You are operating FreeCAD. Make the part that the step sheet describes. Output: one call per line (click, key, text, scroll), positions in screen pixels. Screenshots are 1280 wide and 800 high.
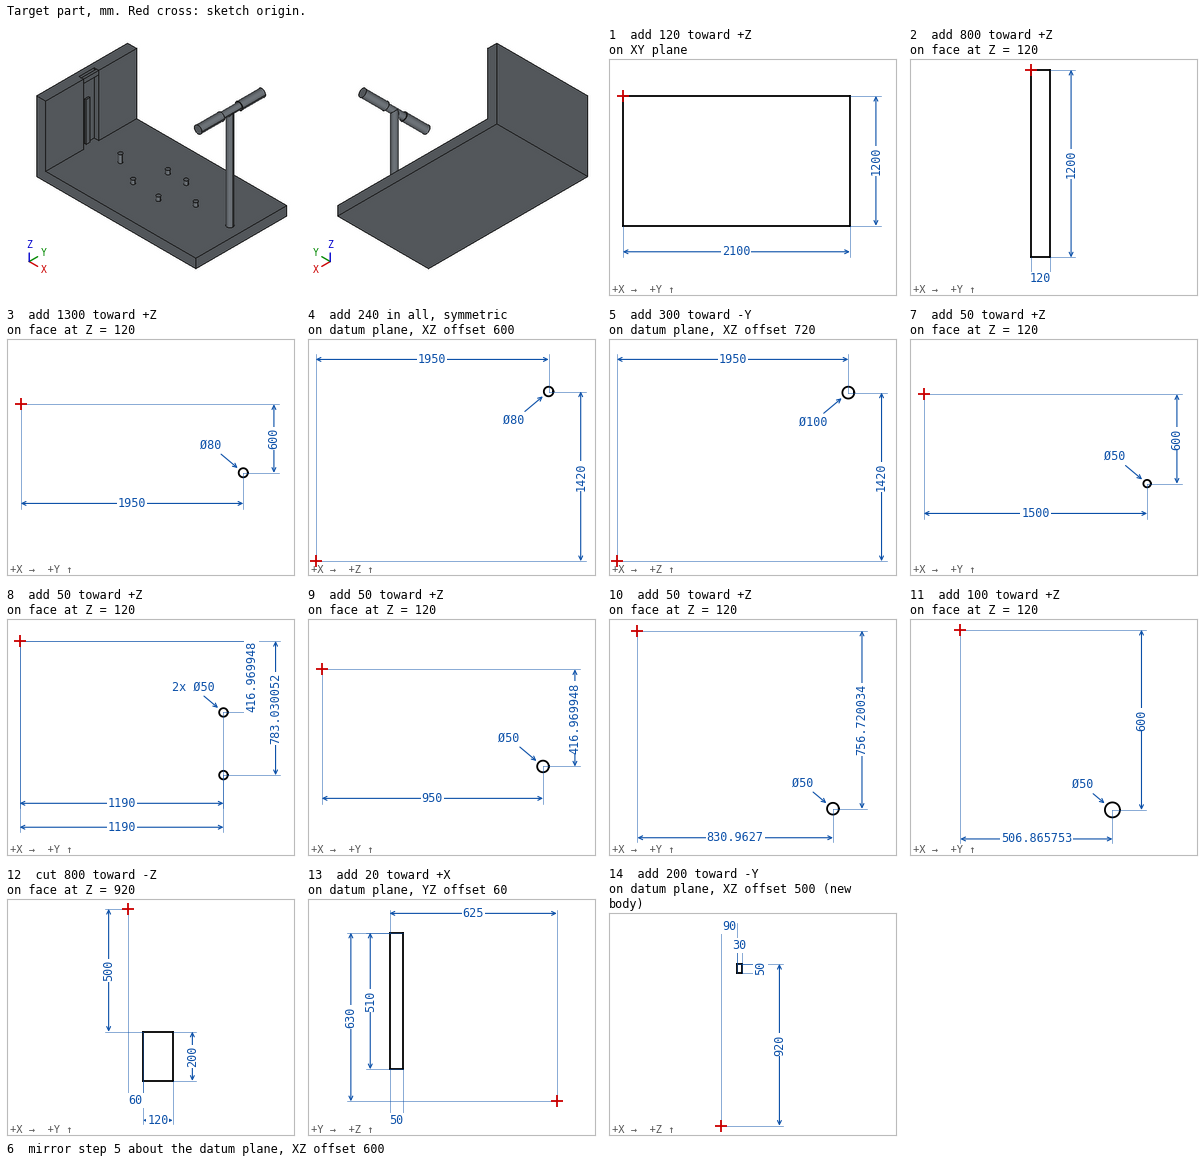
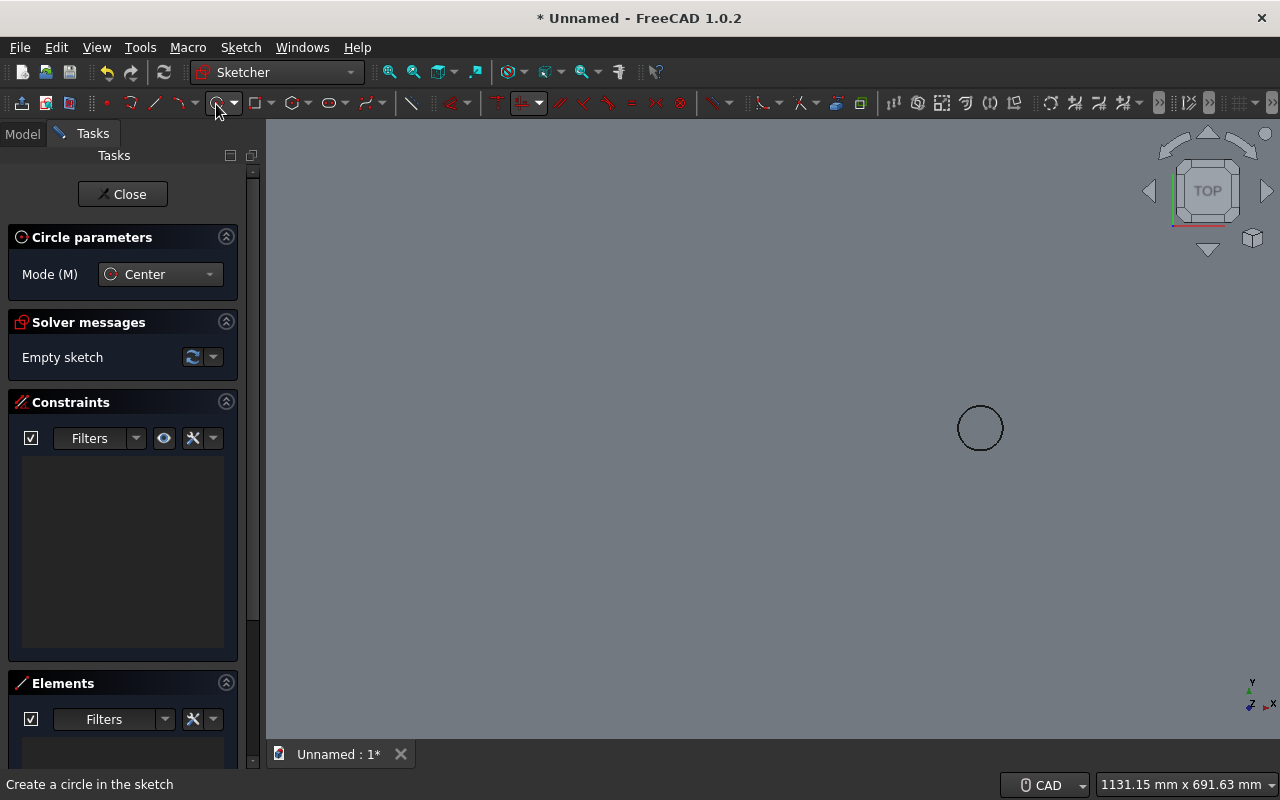
click(703, 264)
move(718, 248)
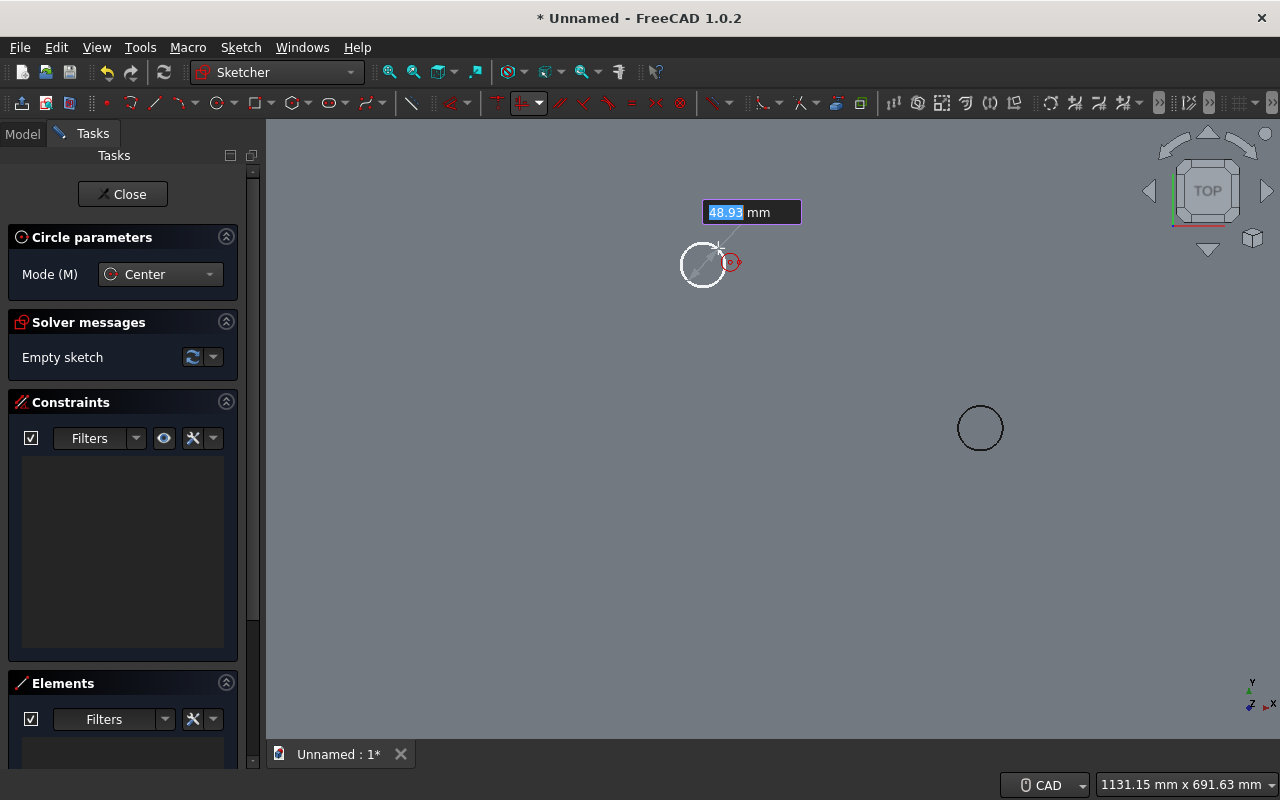
text(50)
key(Return)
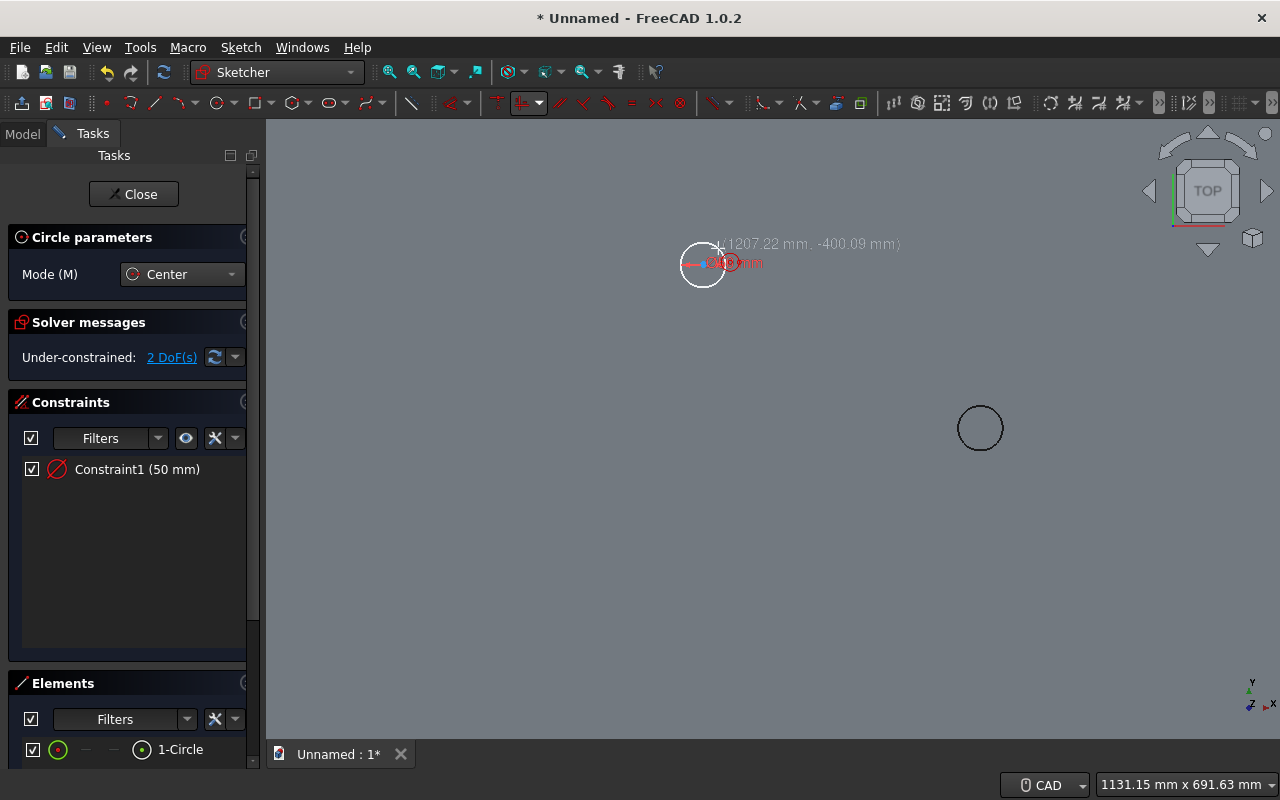
click(703, 592)
move(718, 576)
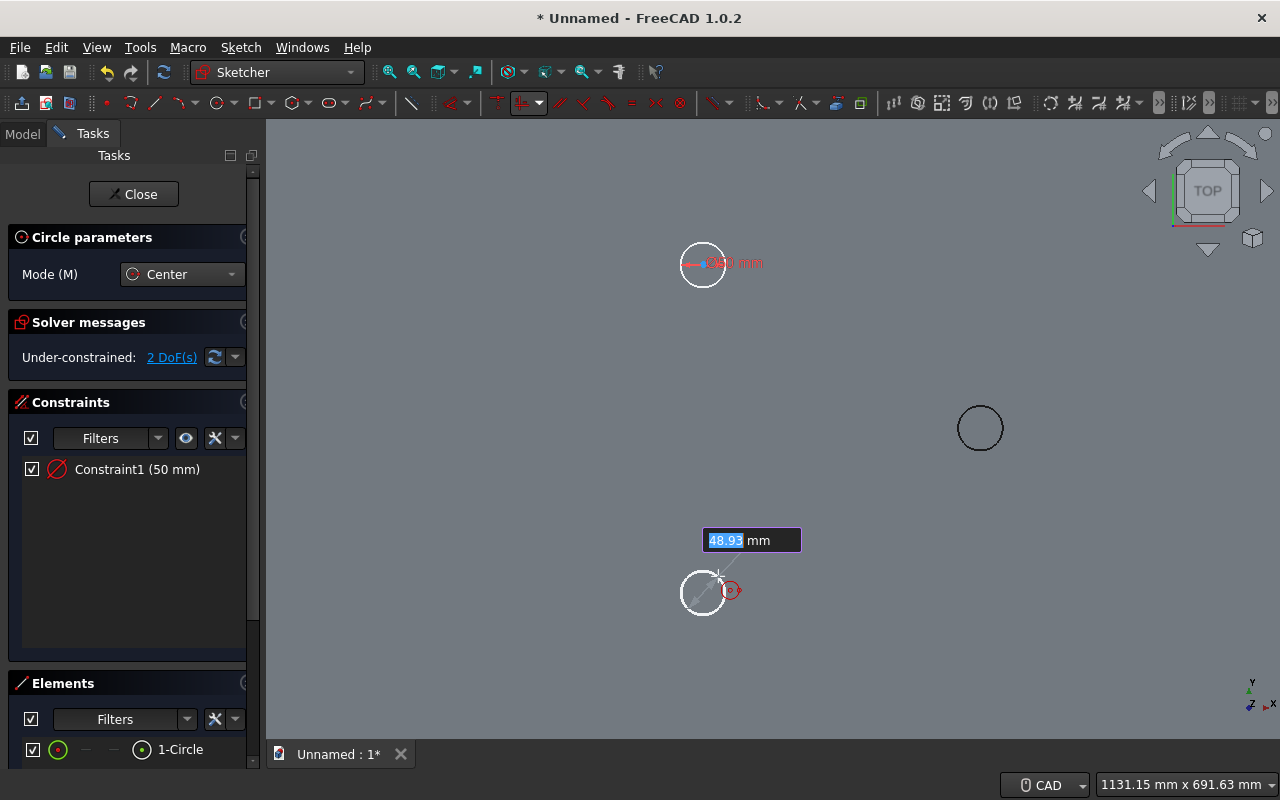
text(50)
key(Return)
key(Escape)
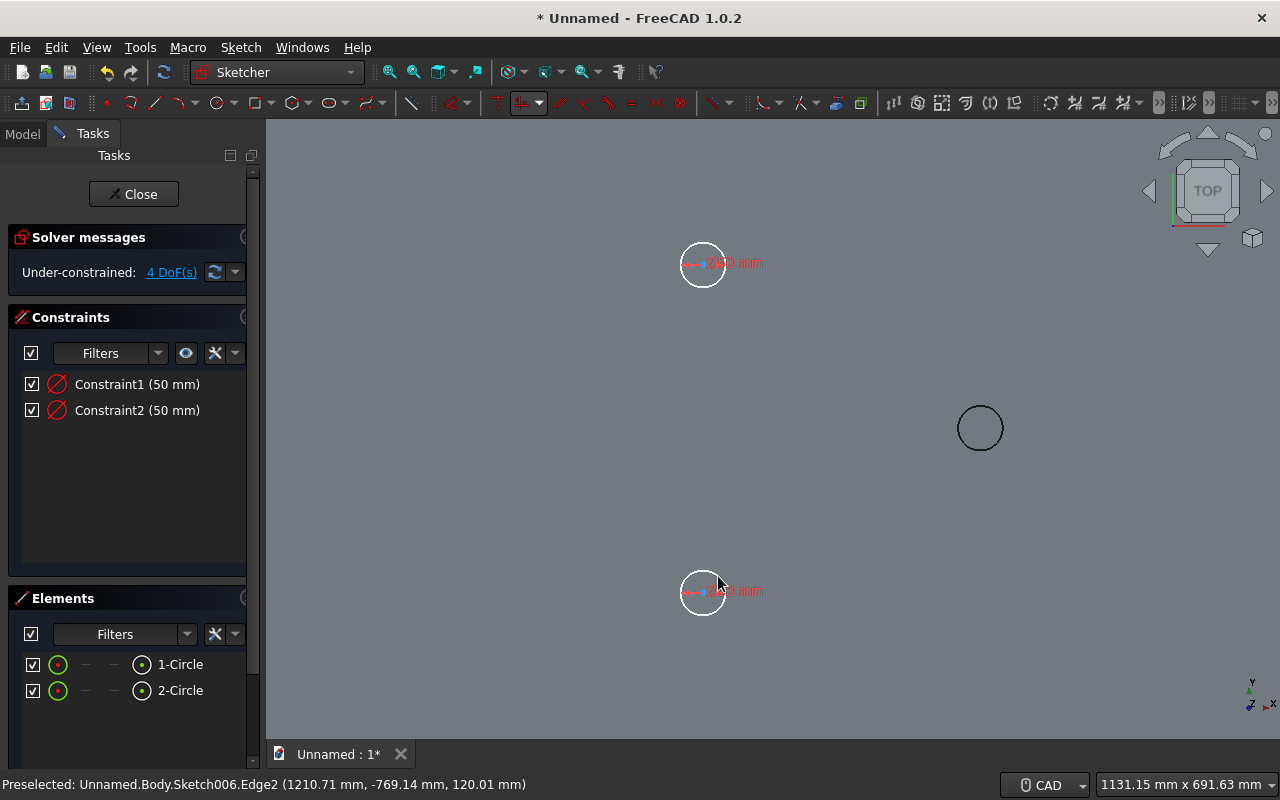
click(450, 104)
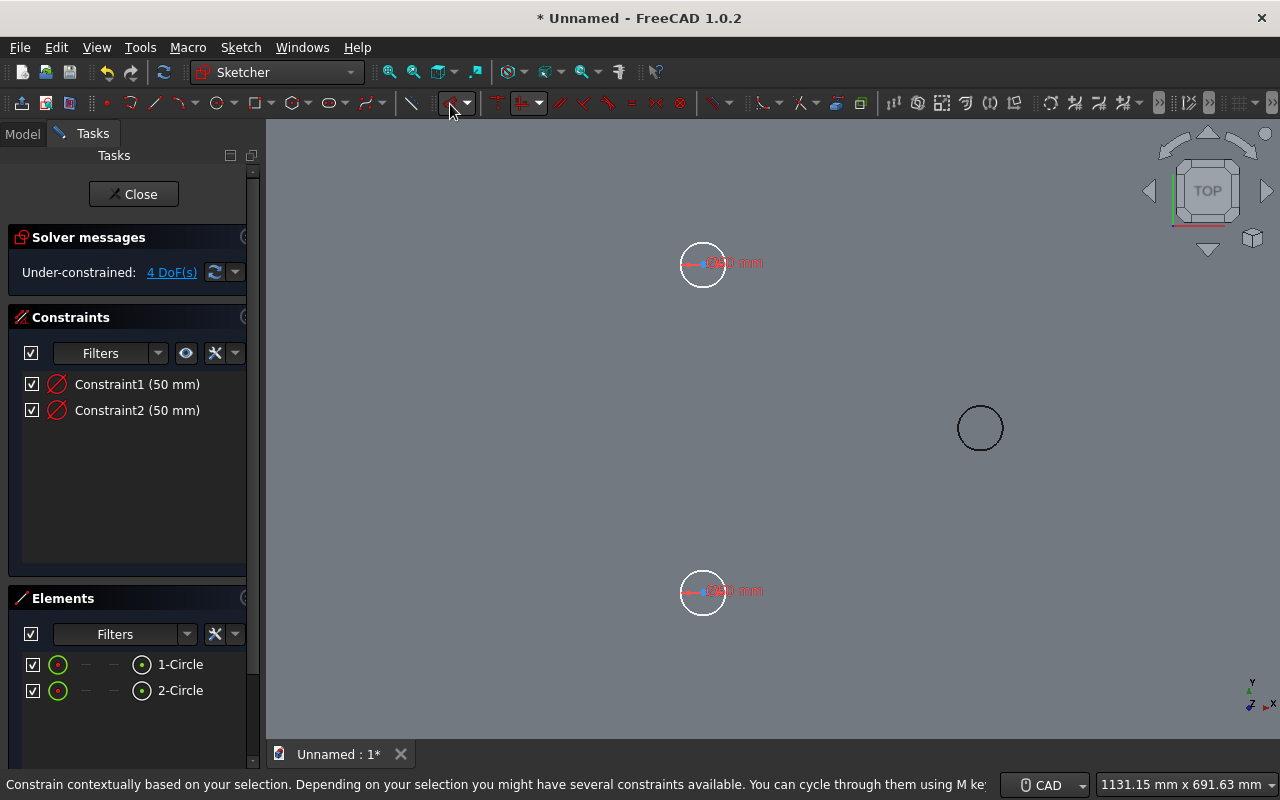
click(703, 265)
click(498, 299)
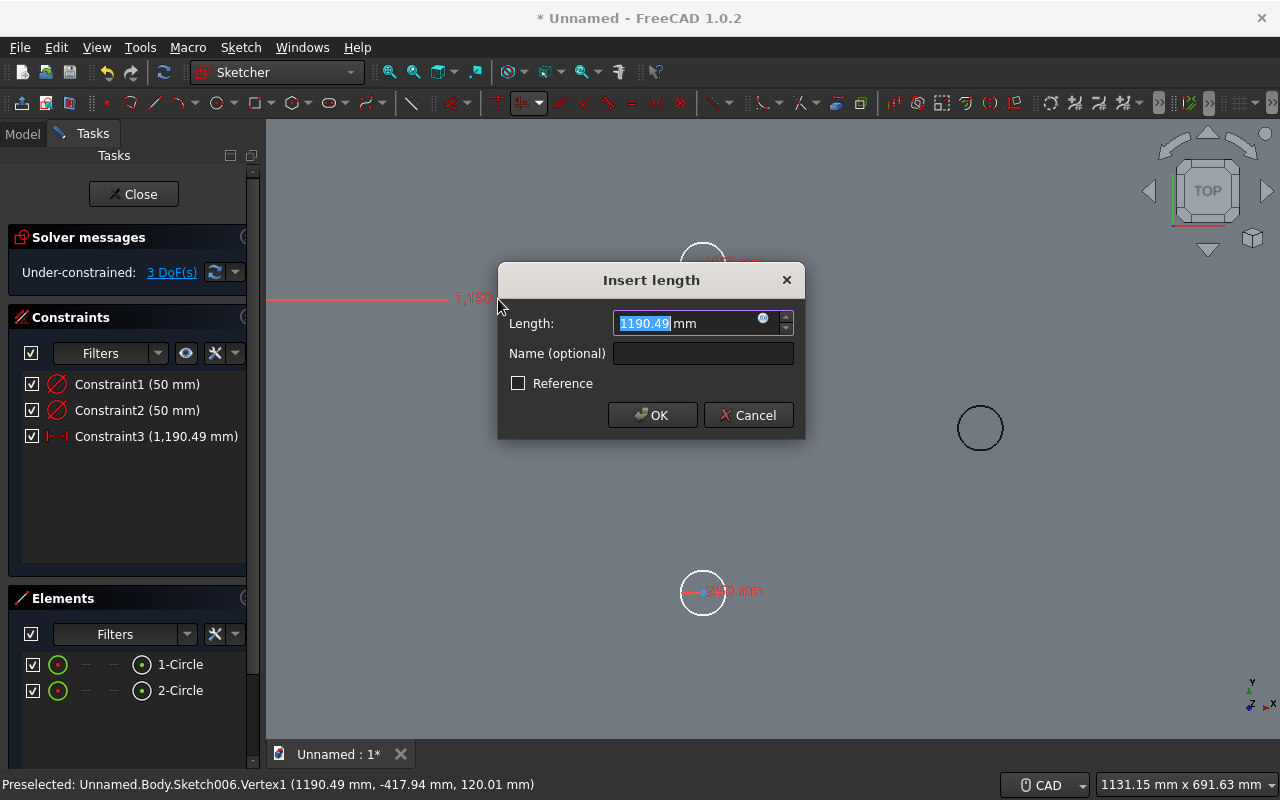
text(1190)
key(Return)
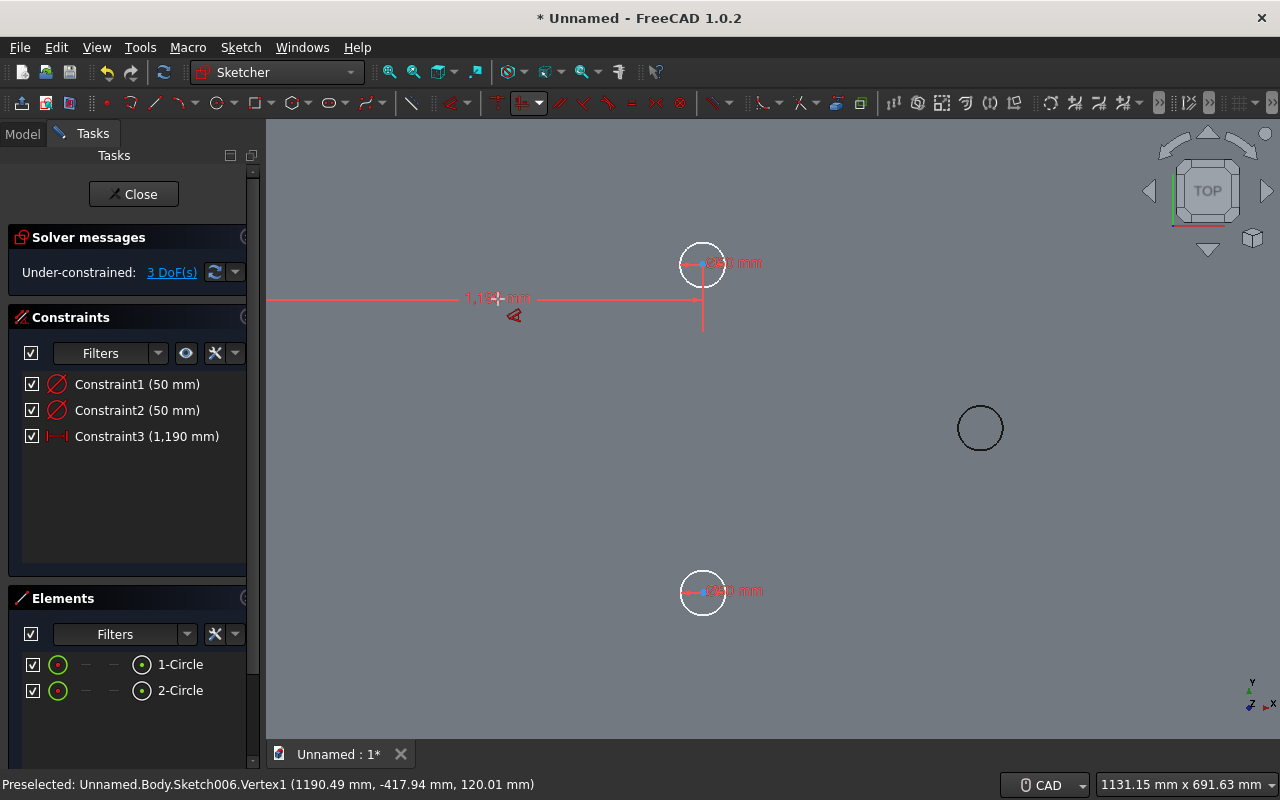
click(703, 593)
click(498, 627)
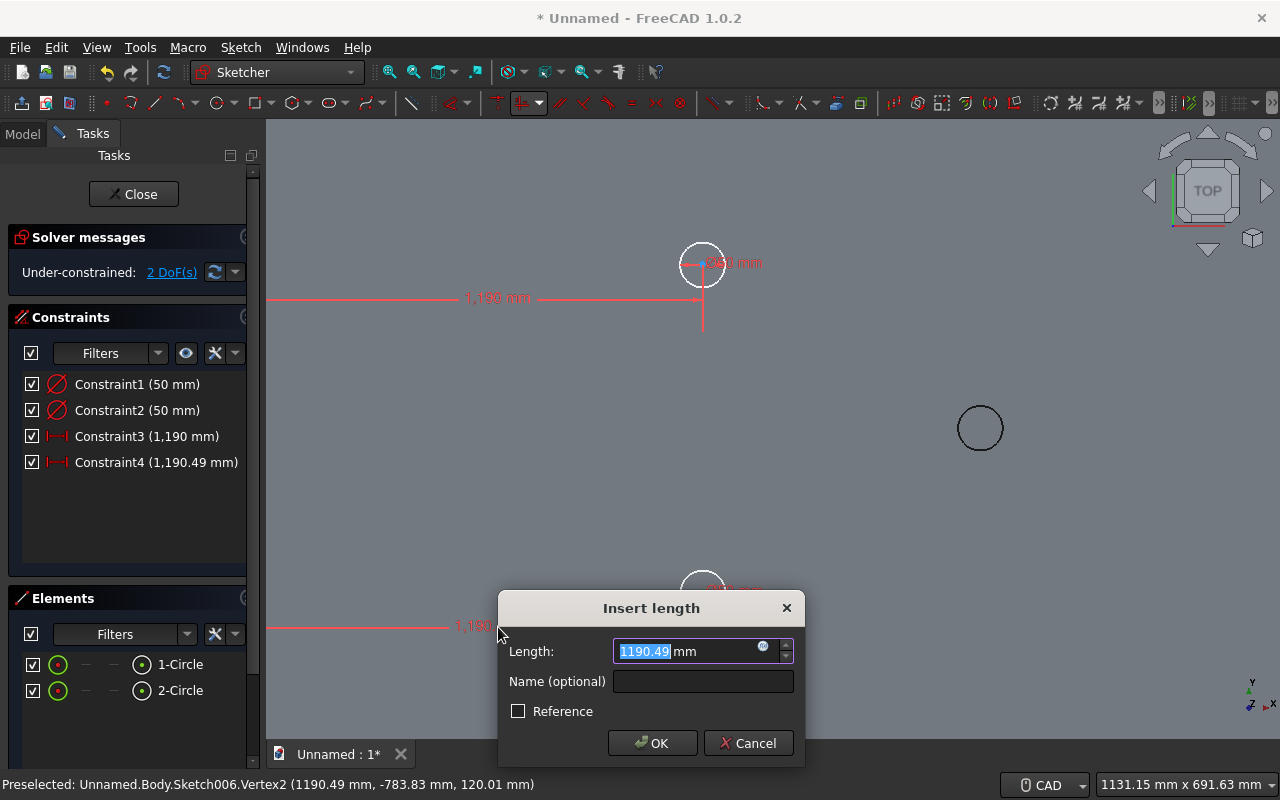
text(1190)
key(Return)